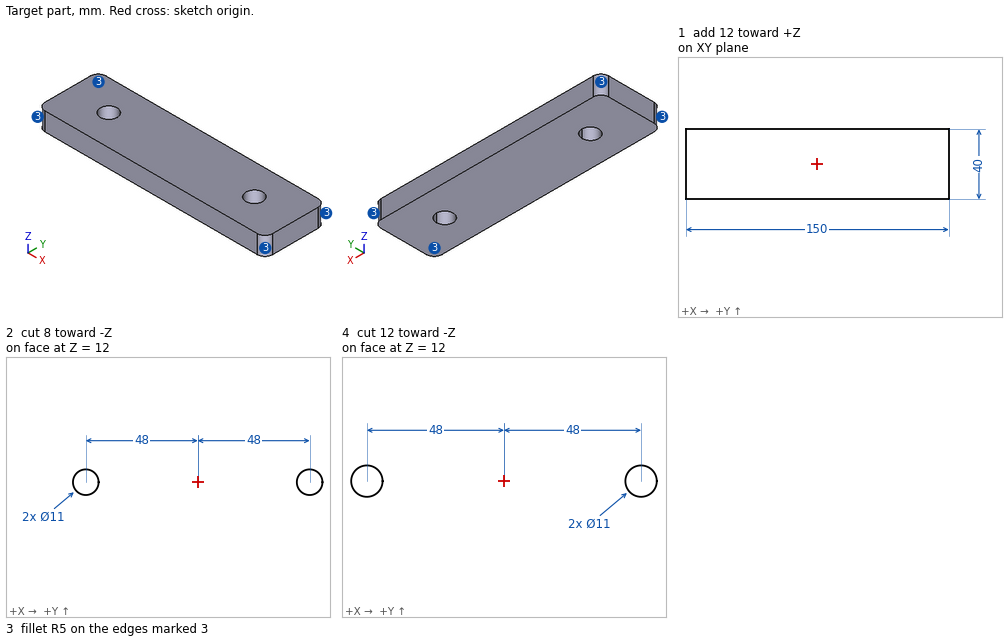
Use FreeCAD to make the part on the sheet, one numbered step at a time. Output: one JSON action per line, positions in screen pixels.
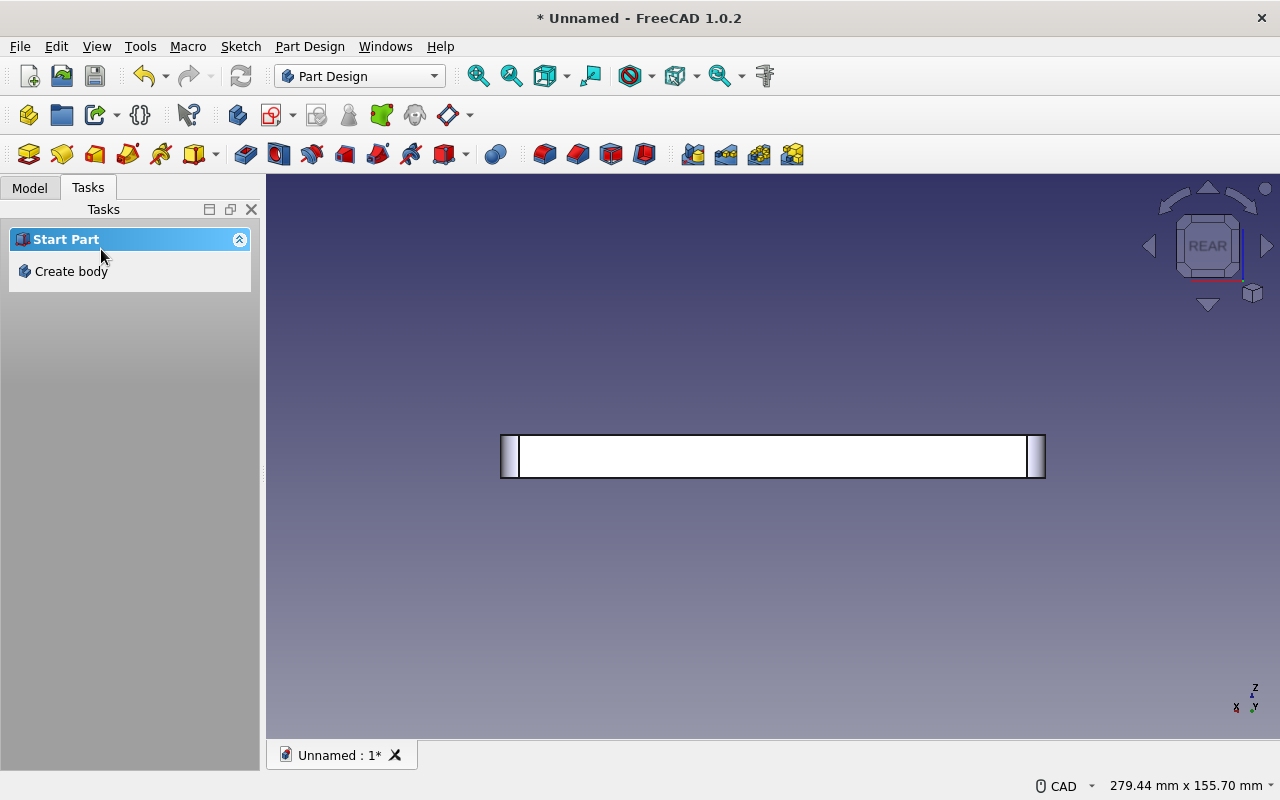
{"action": "key", "text": "0"}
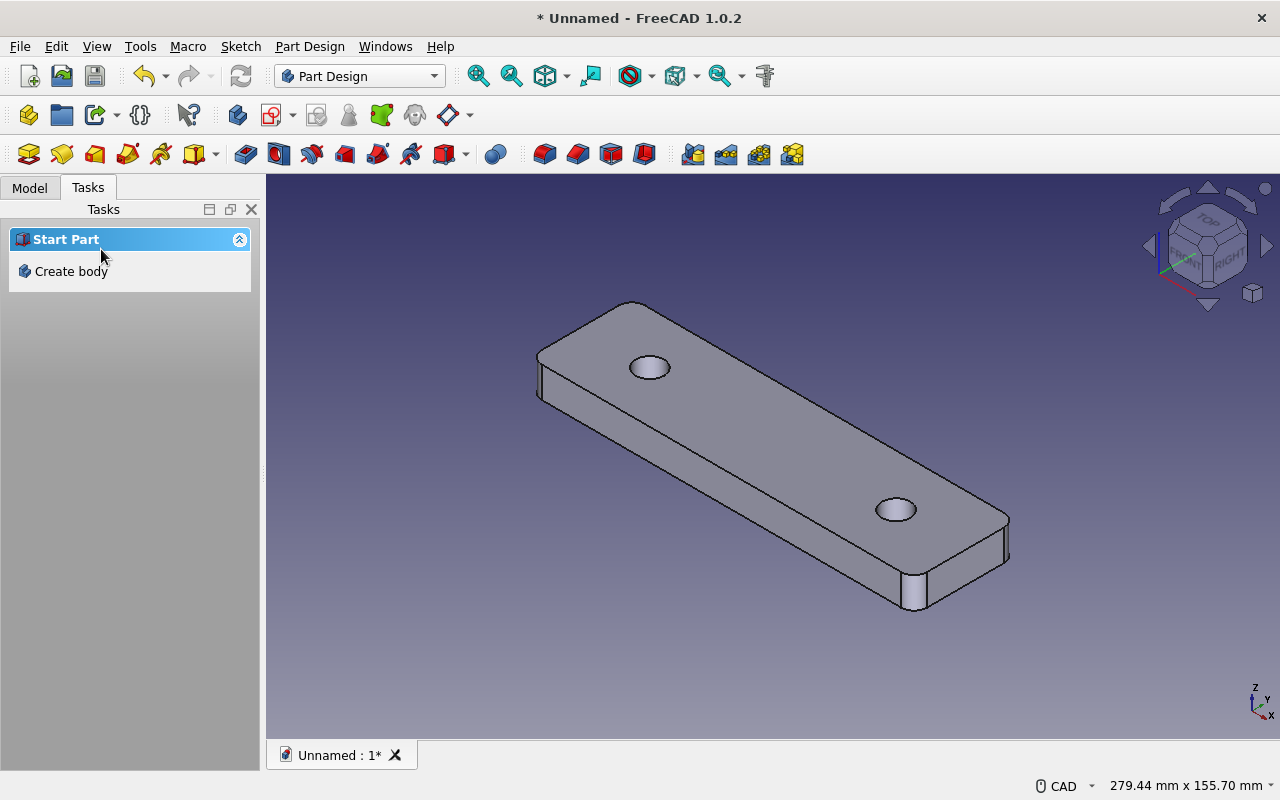
{"action": "left_click", "coordinate": [828, 469]}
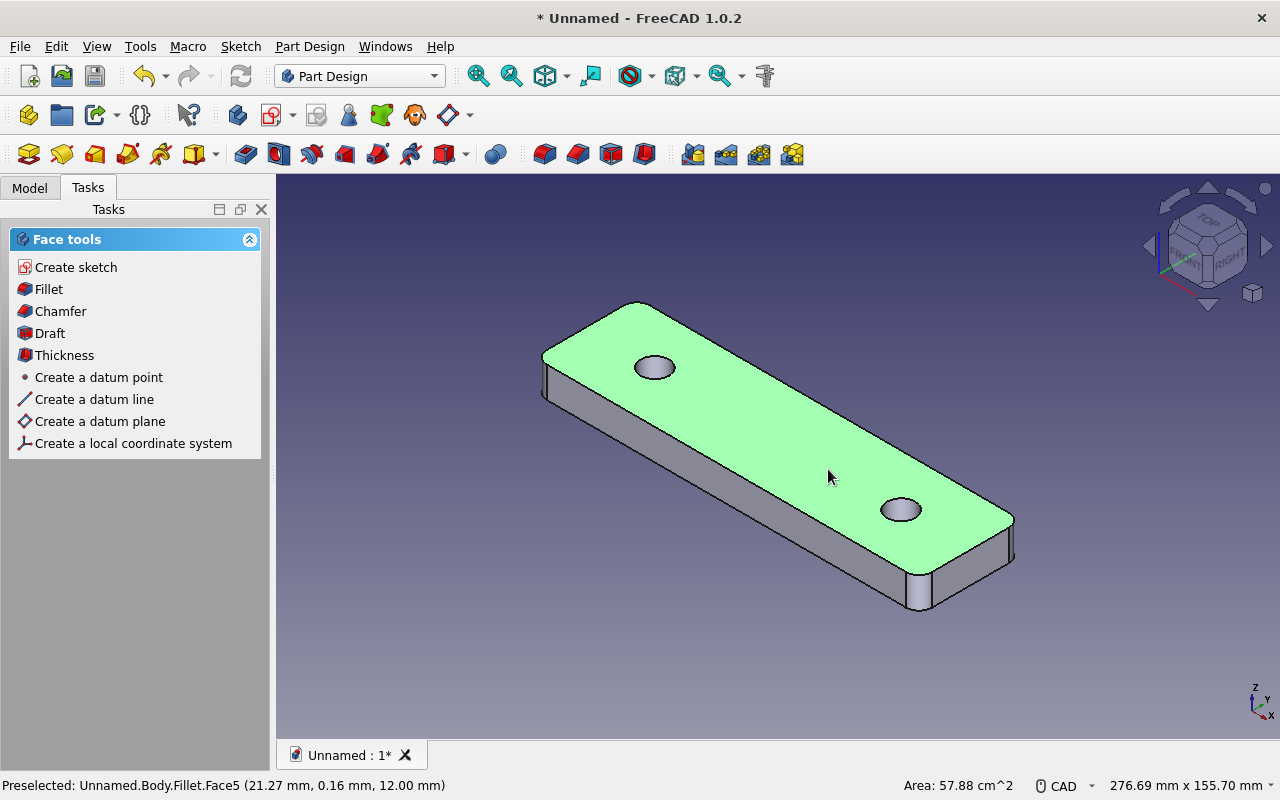
{"action": "left_click", "coordinate": [270, 116]}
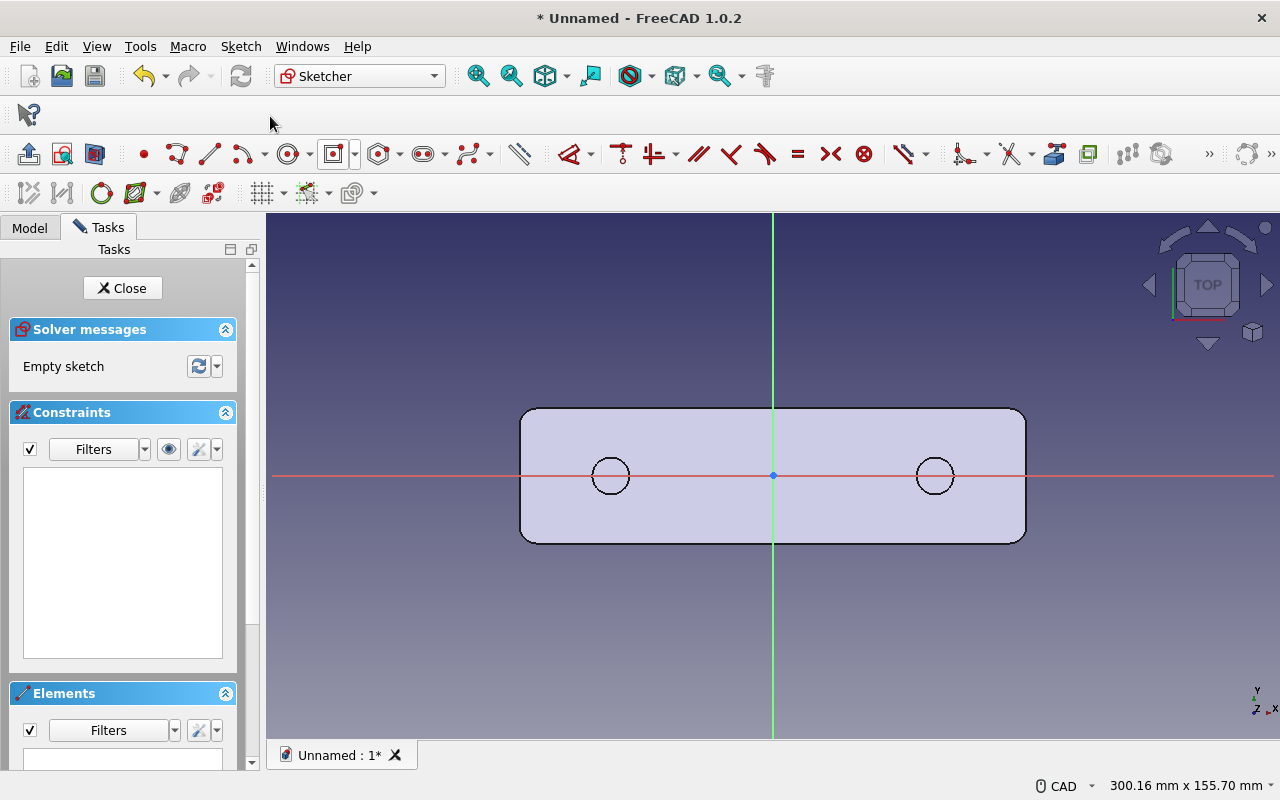
{"action": "scroll", "coordinate": [912, 476], "scroll_direction": "up", "scroll_amount": 2}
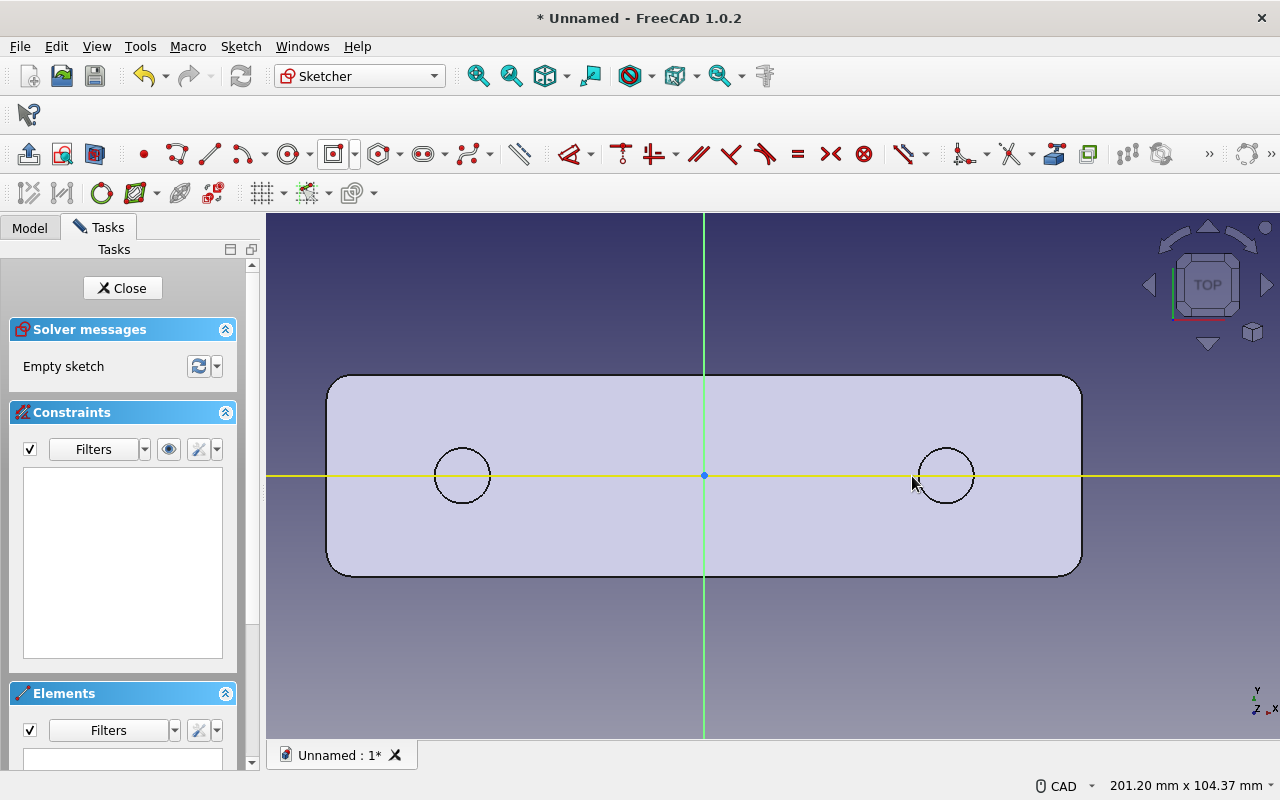
{"action": "left_click", "coordinate": [288, 154]}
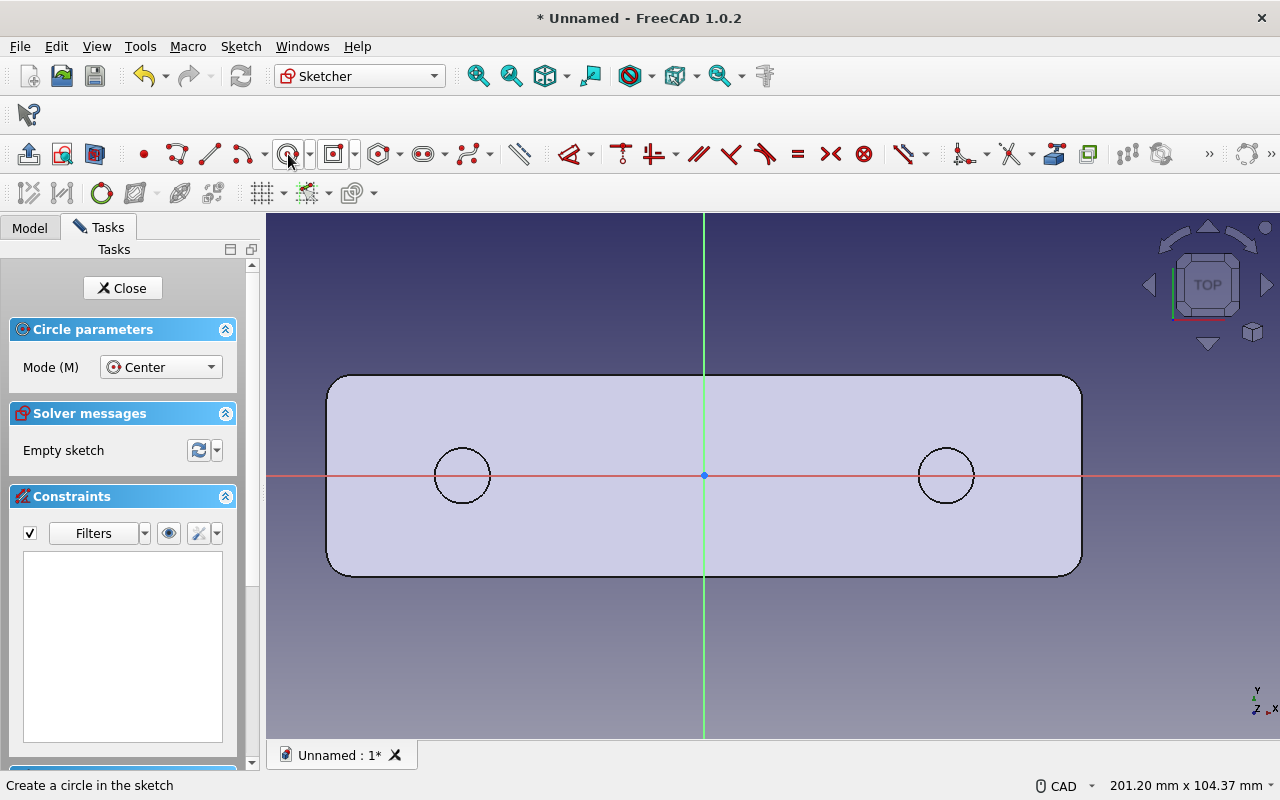
{"action": "left_click", "coordinate": [946, 476]}
{"action": "left_click", "coordinate": [966, 456]}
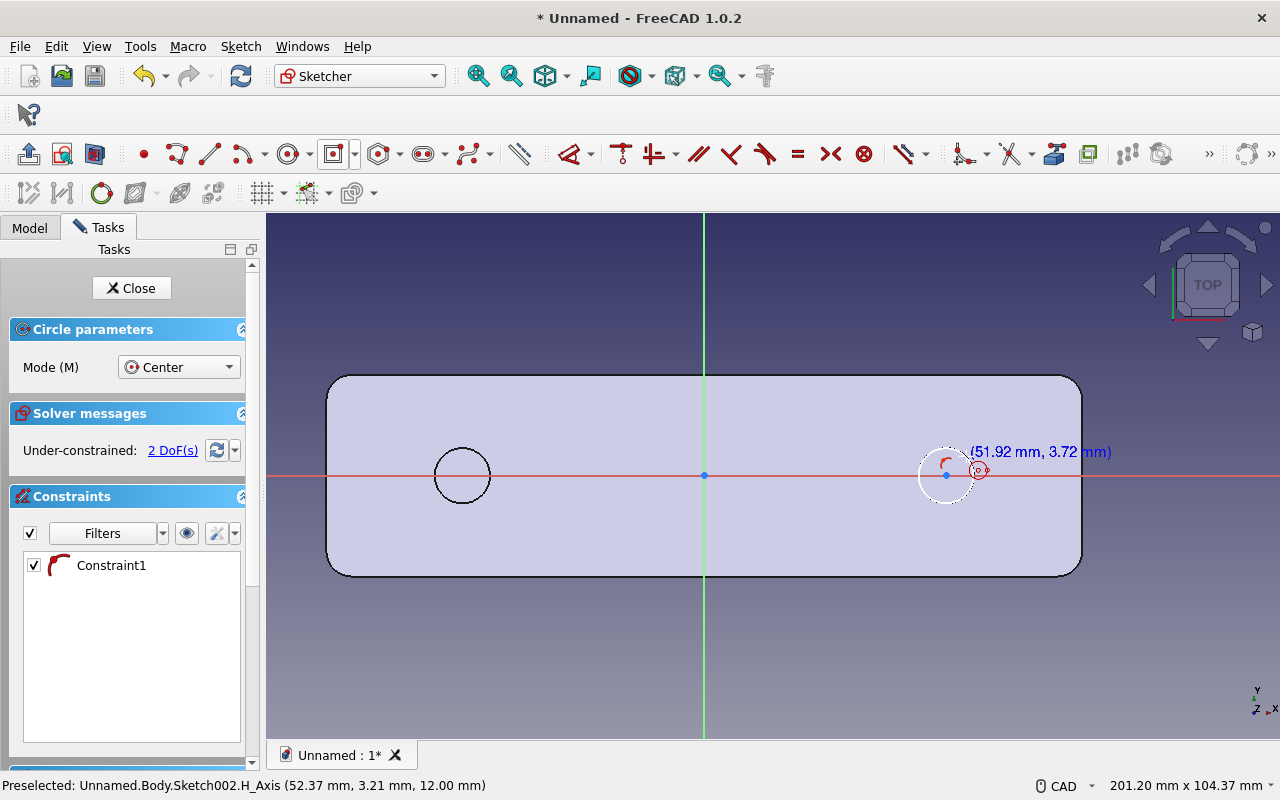
{"action": "left_click", "coordinate": [462, 476]}
{"action": "left_click", "coordinate": [482, 456]}
{"action": "key", "text": "Escape"}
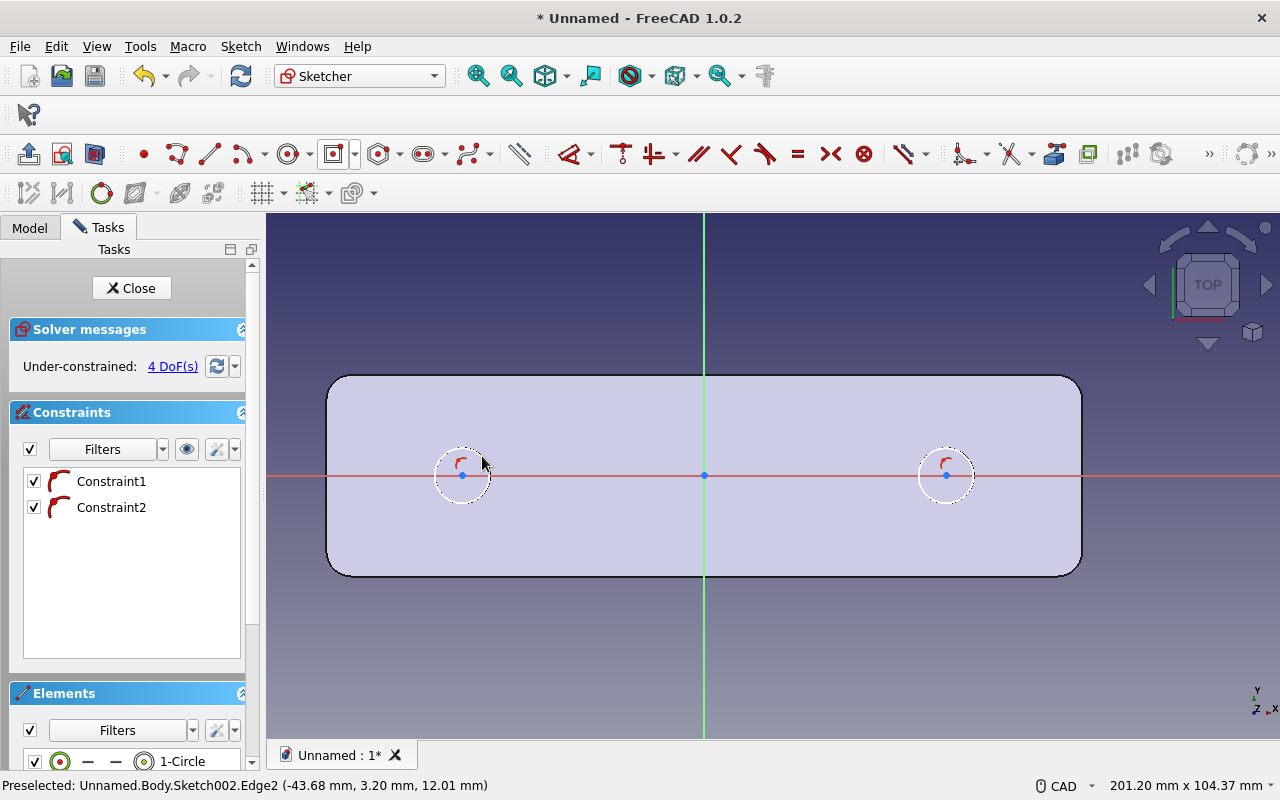
{"action": "left_click", "coordinate": [965, 456]}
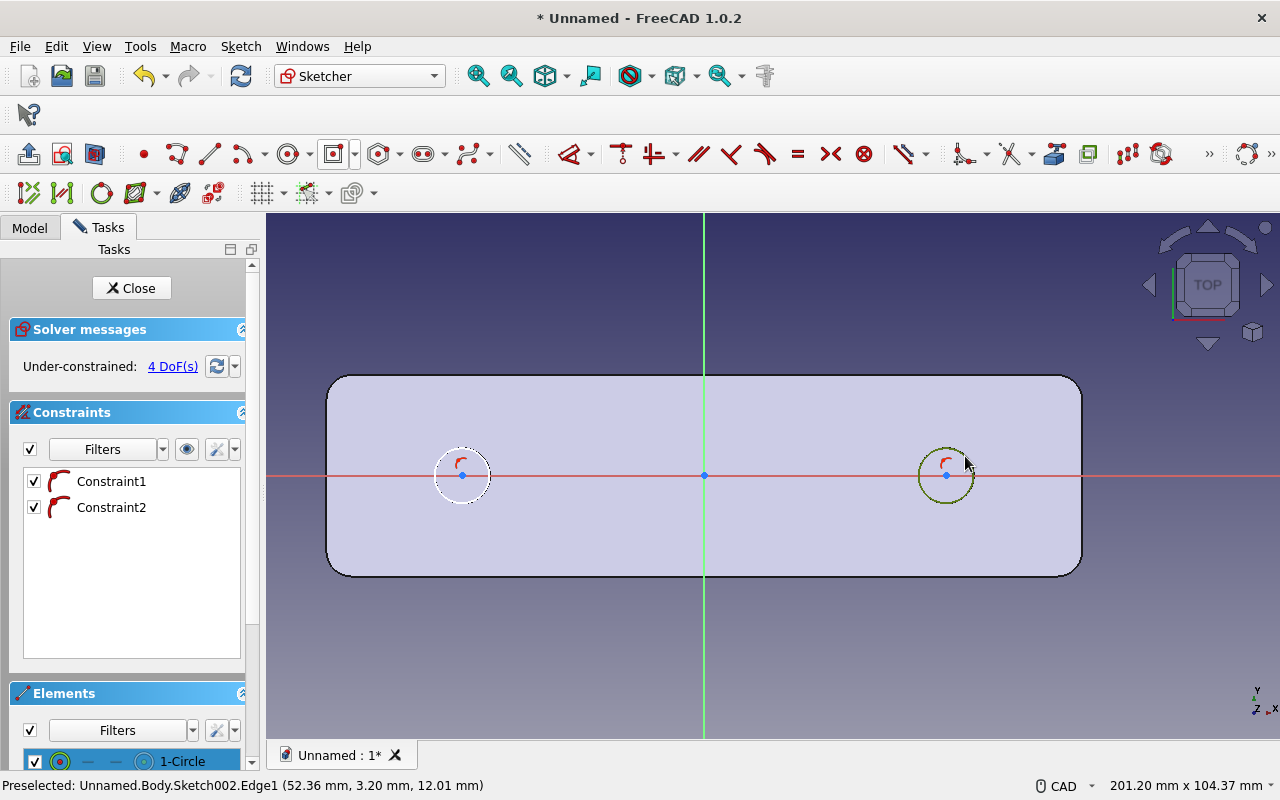
{"action": "left_click", "coordinate": [481, 456]}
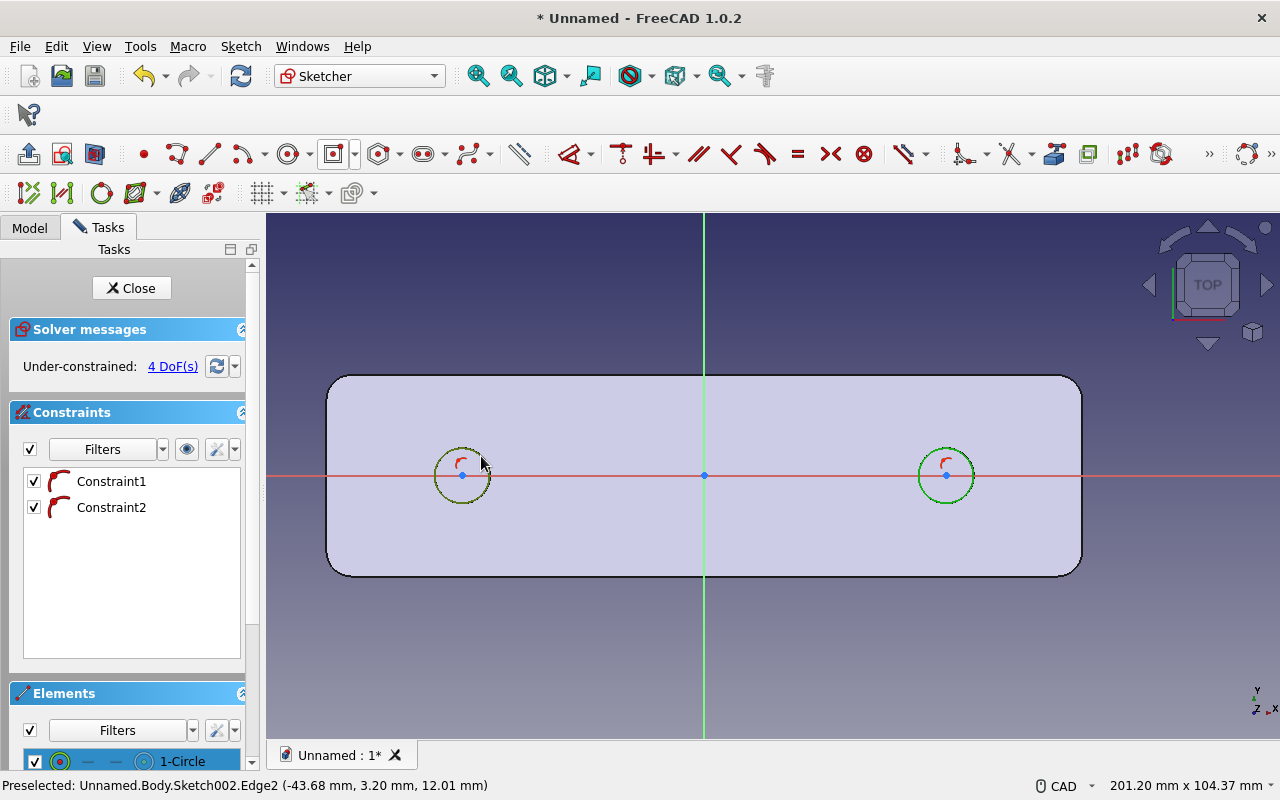
{"action": "left_click", "coordinate": [798, 154]}